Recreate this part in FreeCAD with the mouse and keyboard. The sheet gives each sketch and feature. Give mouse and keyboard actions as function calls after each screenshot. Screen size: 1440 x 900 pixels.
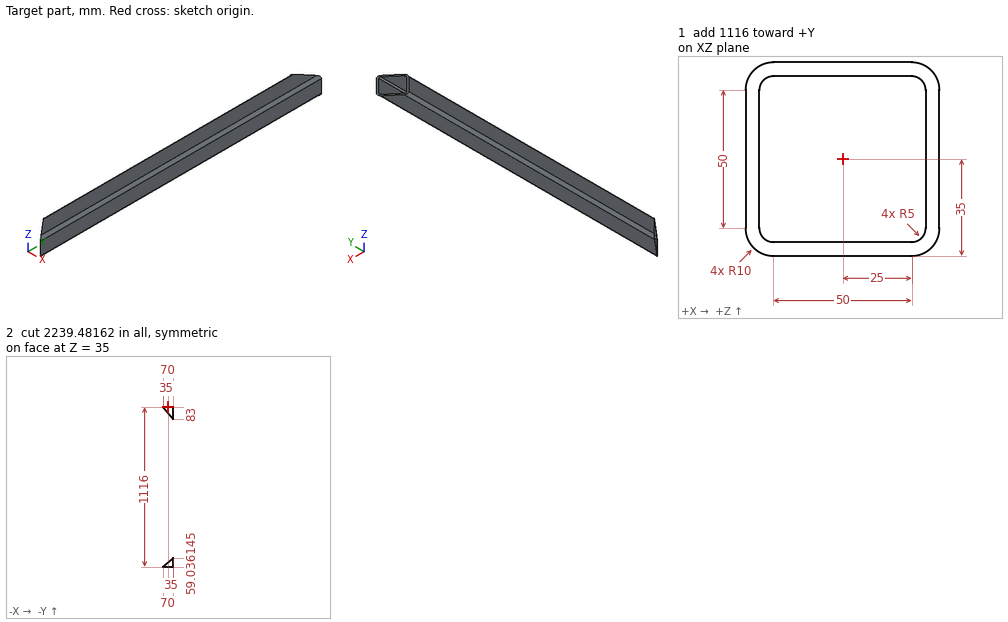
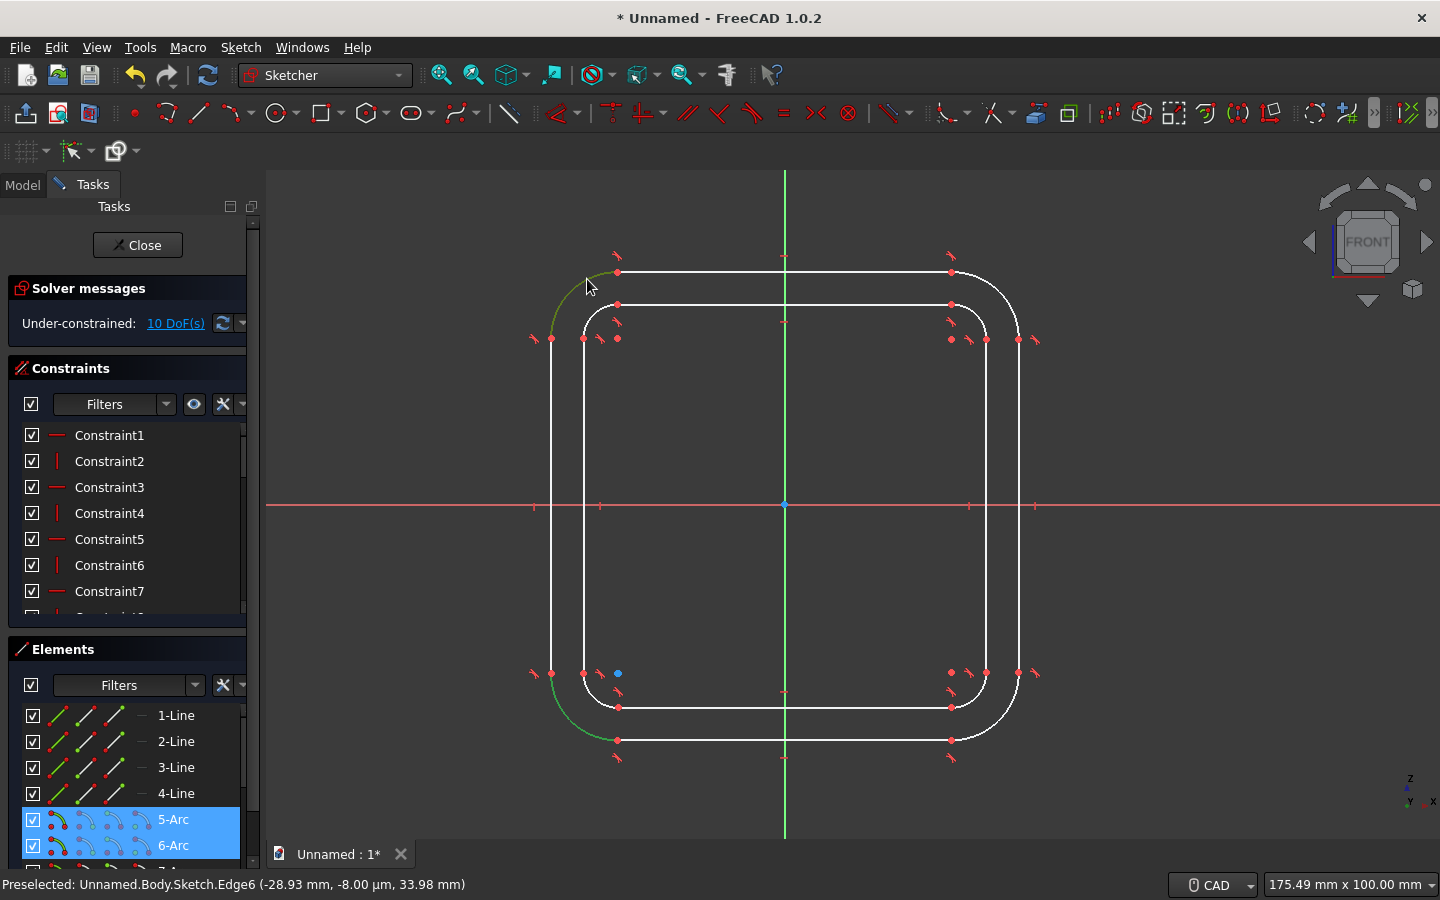
click(1012, 309)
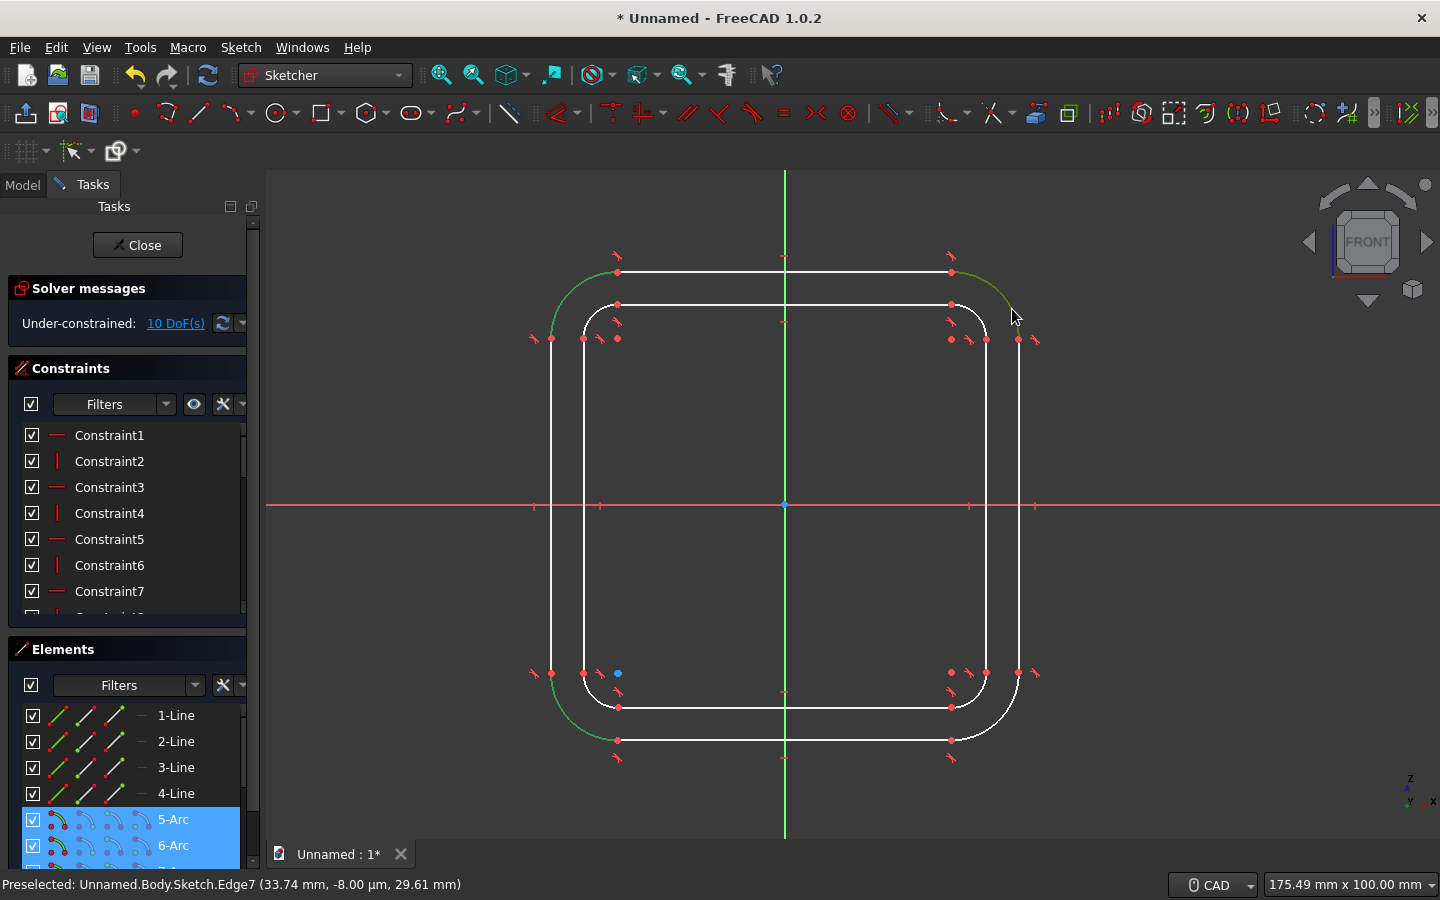
click(982, 733)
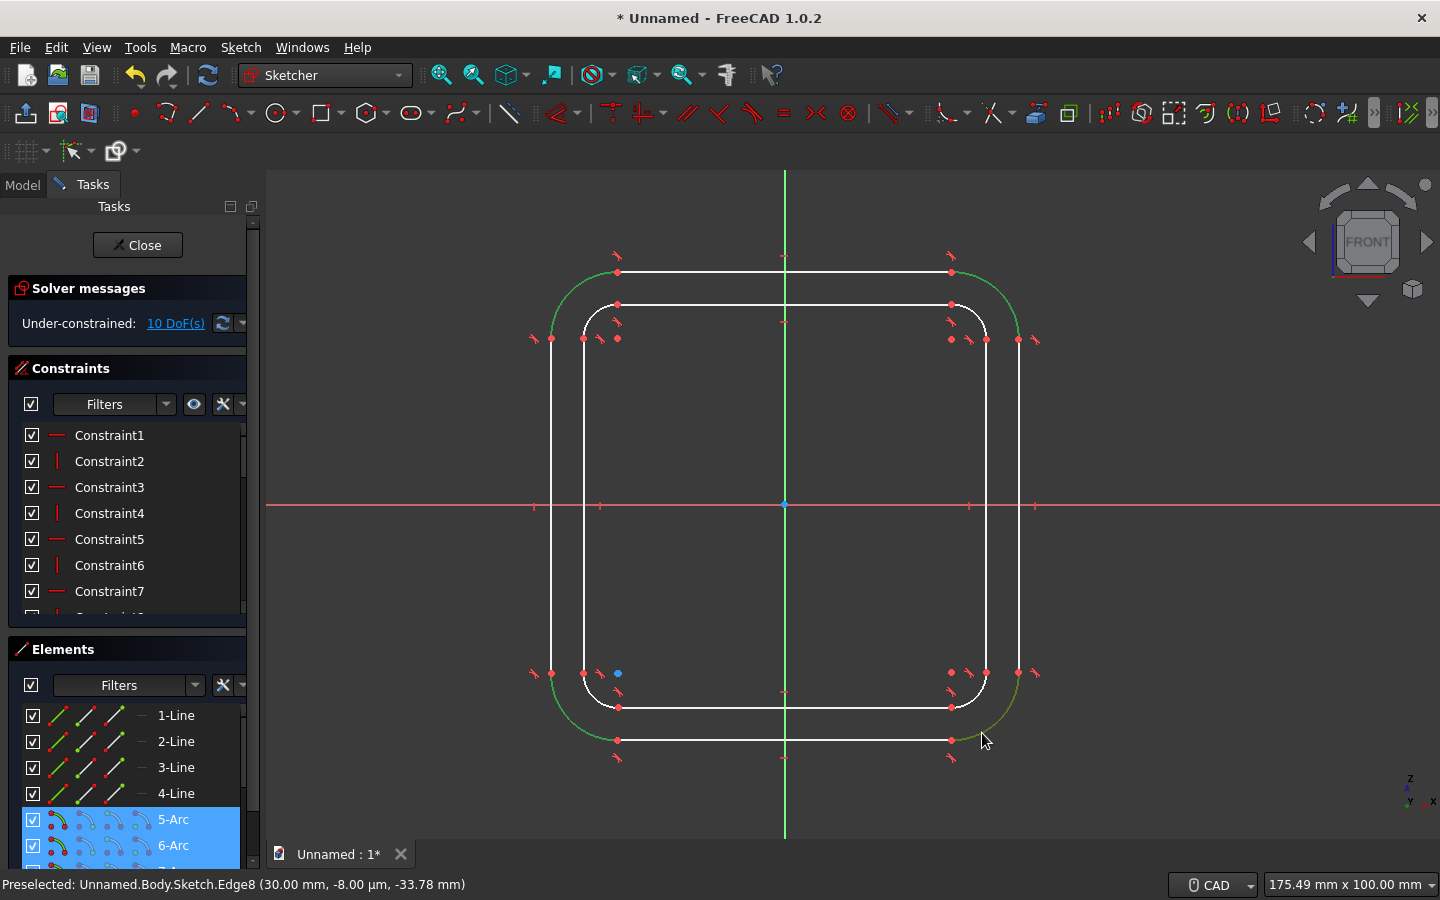
click(784, 114)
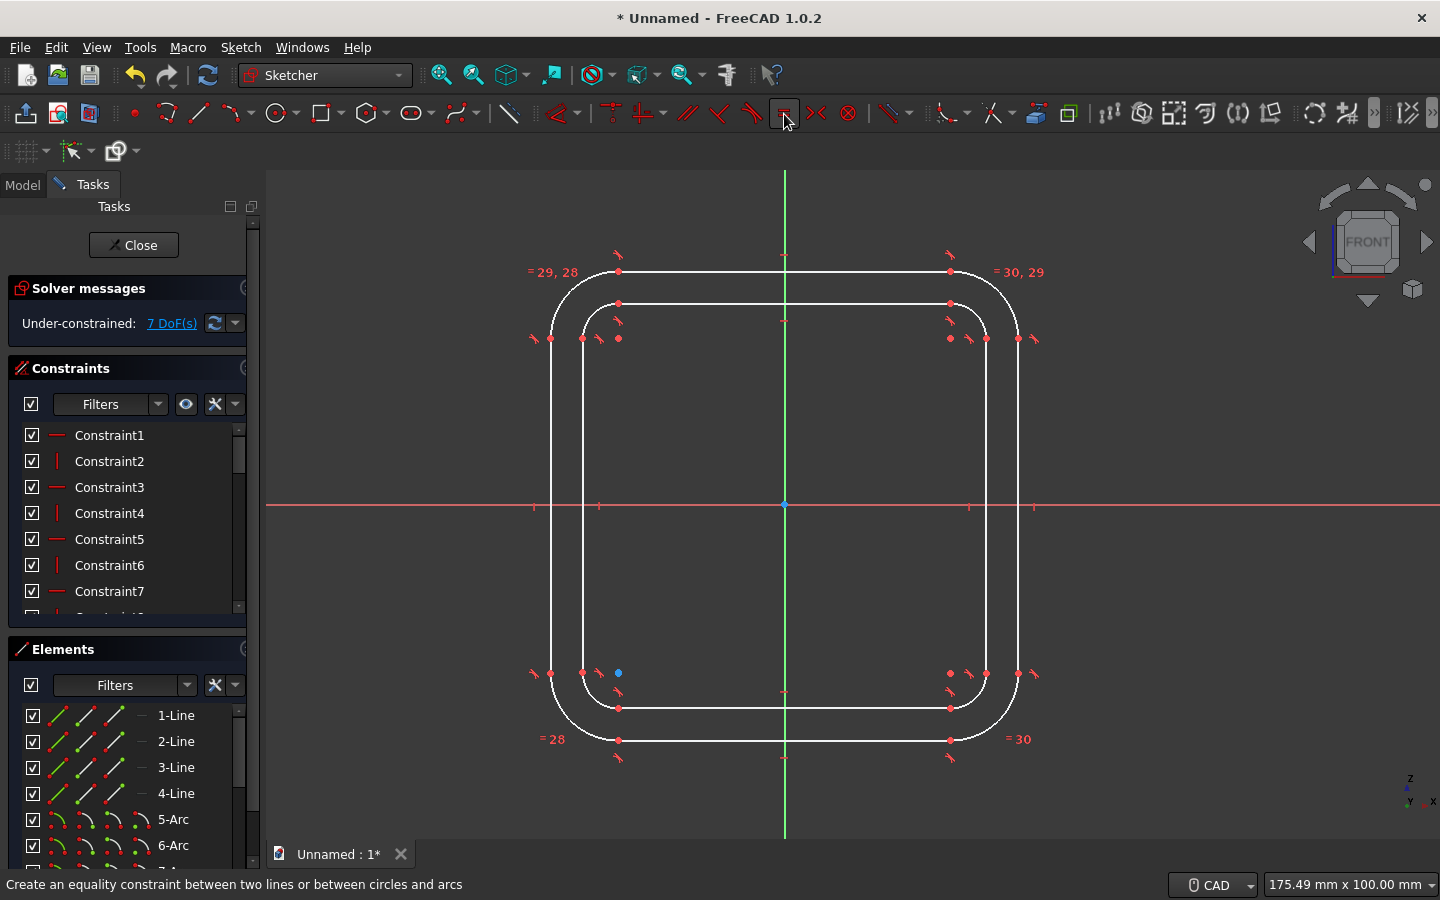
click(967, 705)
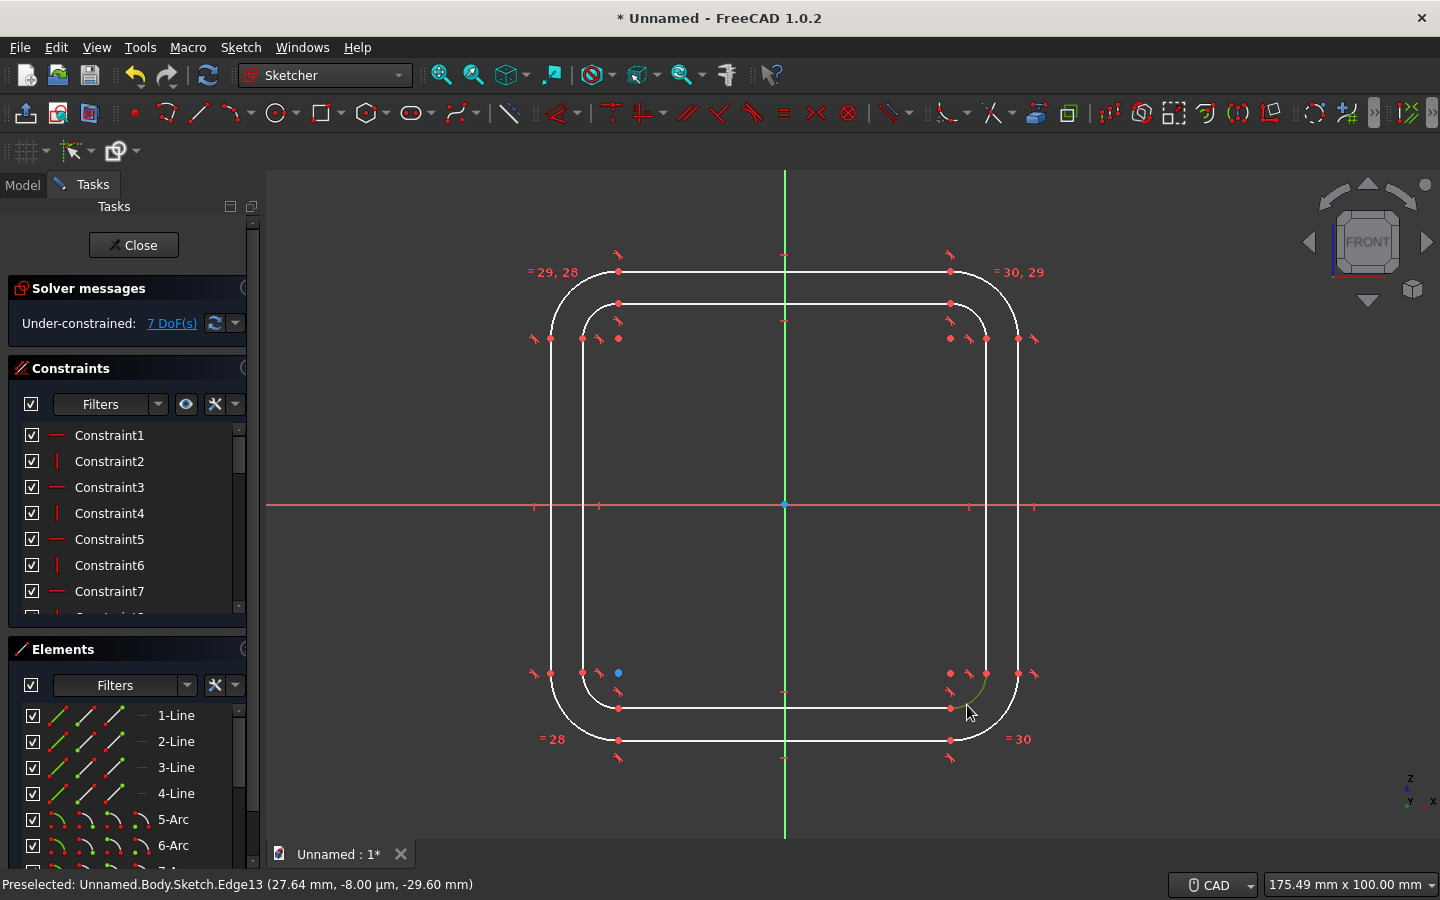
click(587, 689)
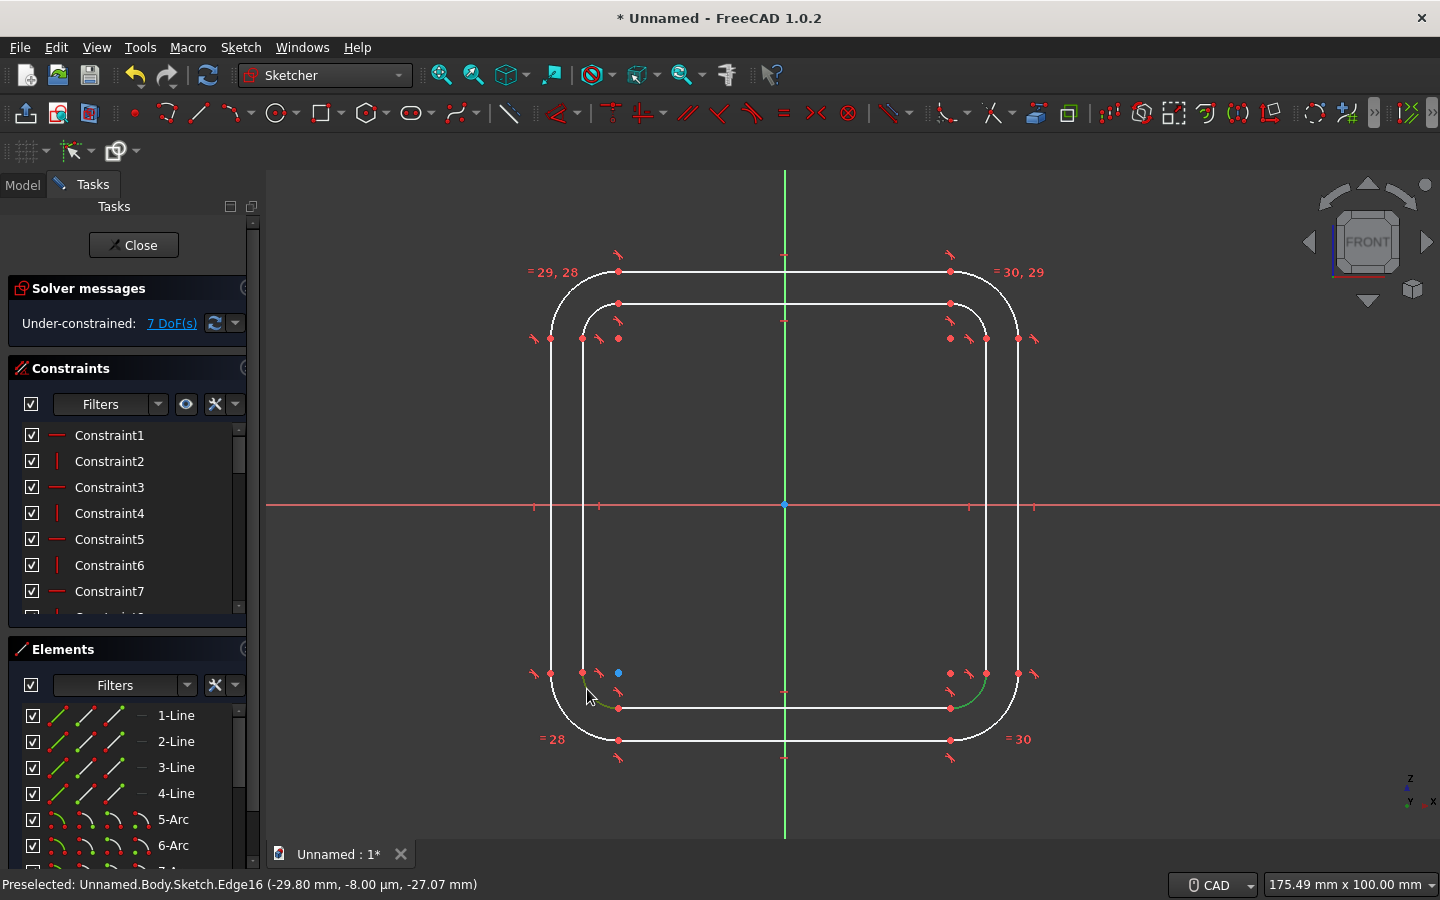
click(784, 114)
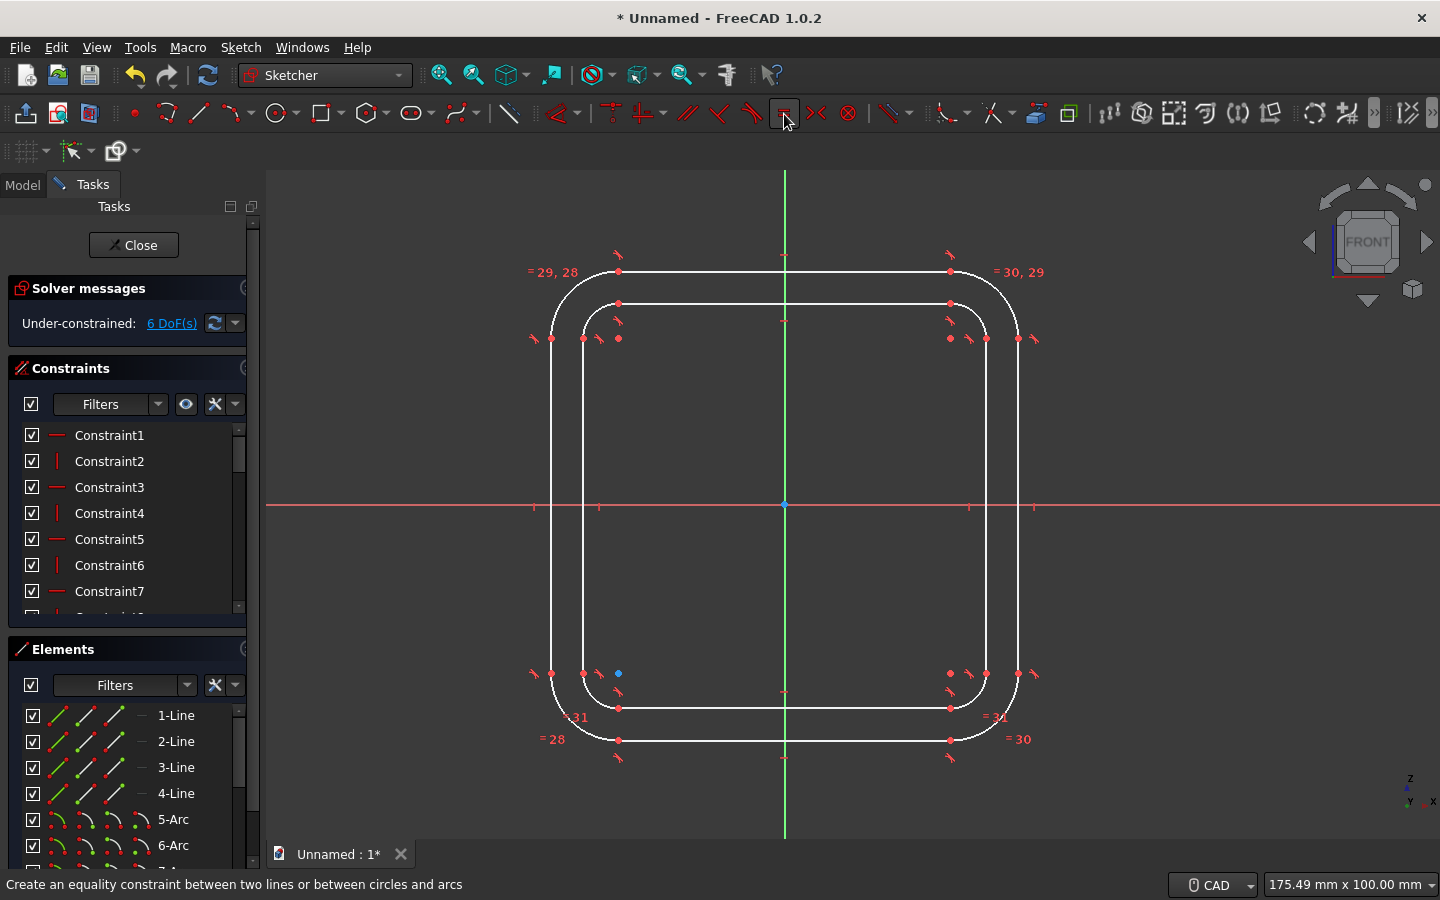
click(556, 114)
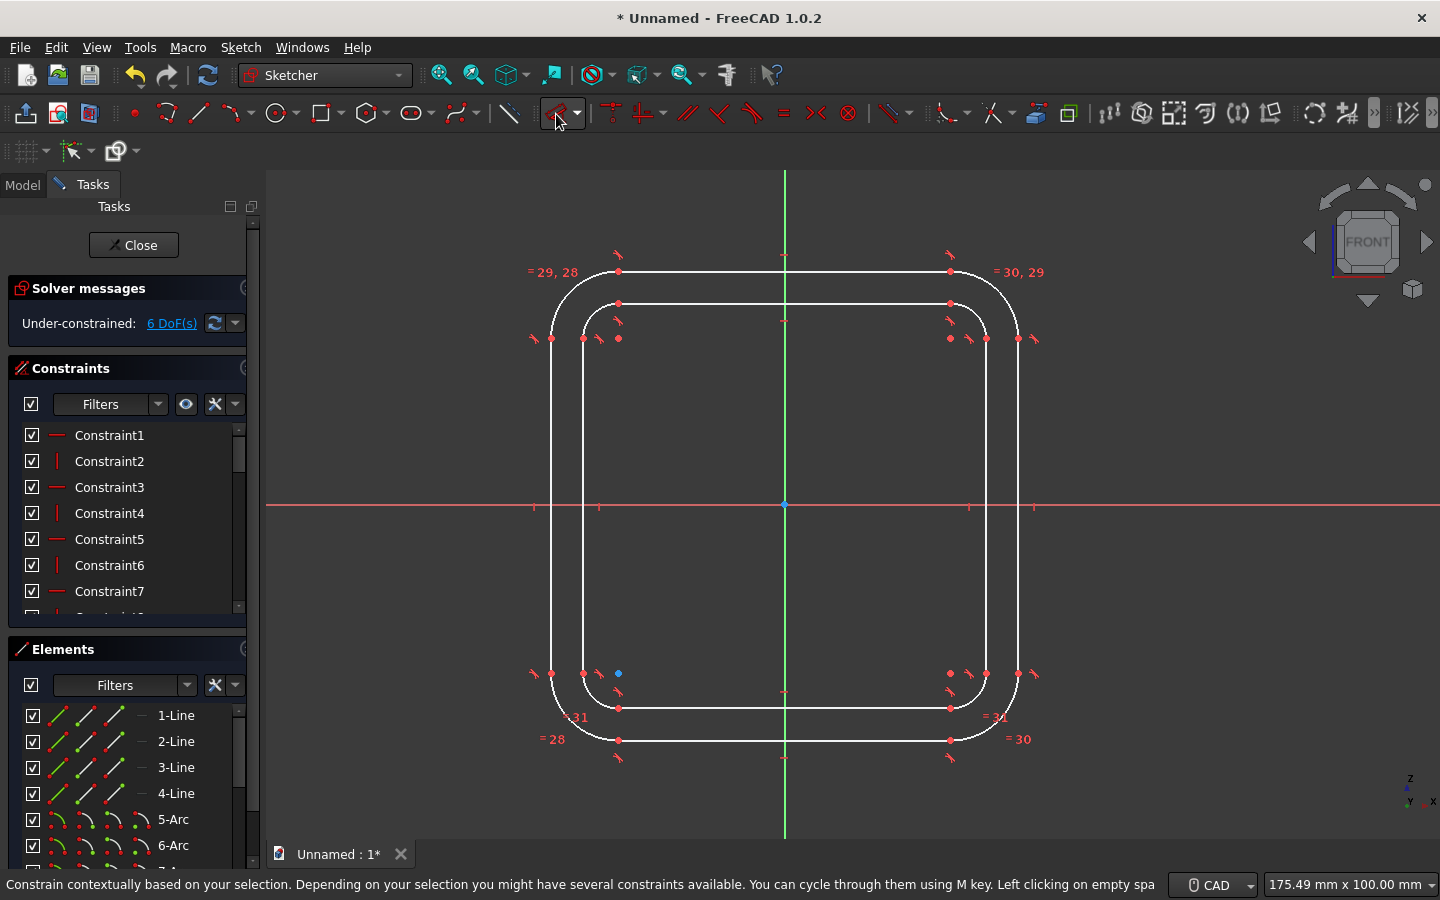
click(558, 704)
click(530, 719)